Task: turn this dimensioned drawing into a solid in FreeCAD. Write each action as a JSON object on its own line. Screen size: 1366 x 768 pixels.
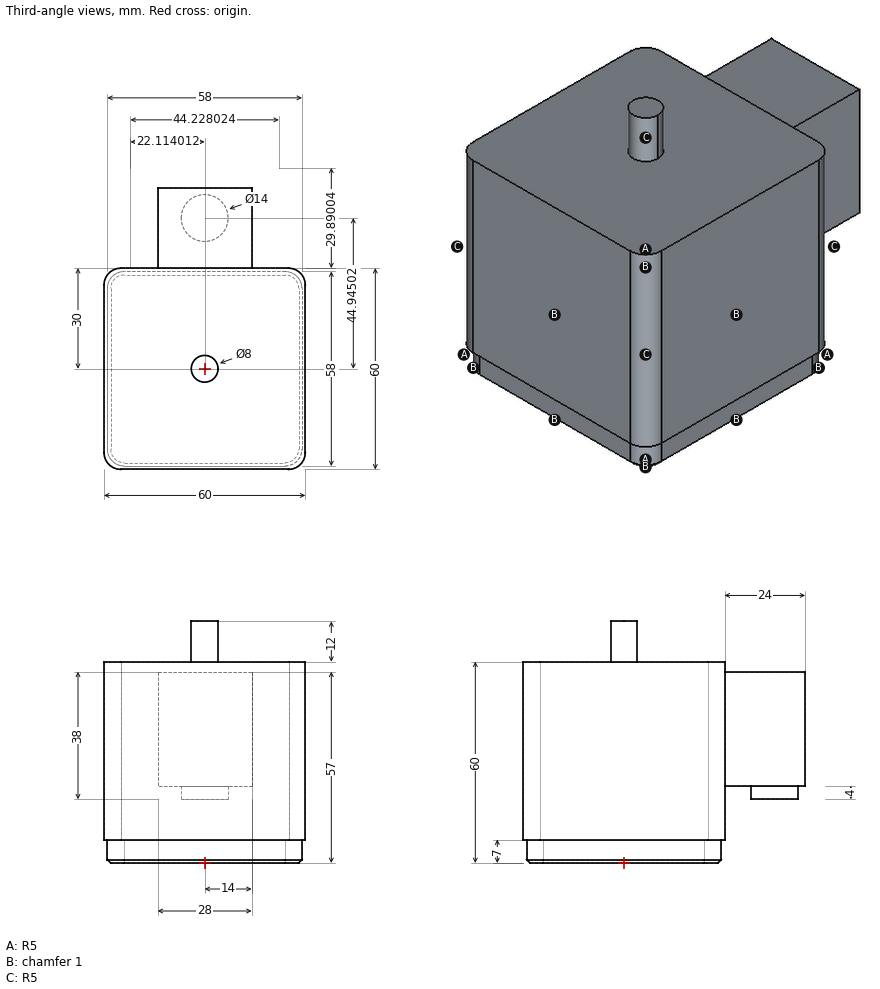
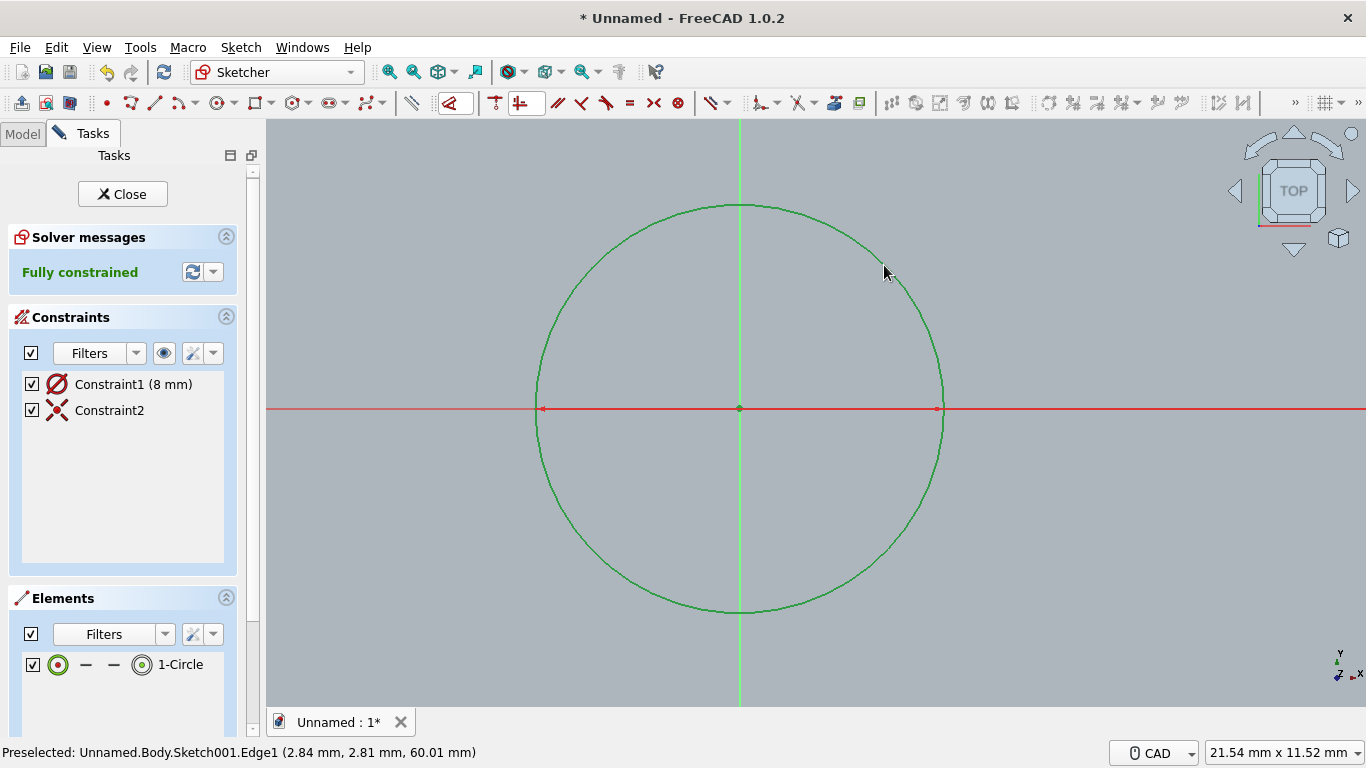
{"action": "left_click", "coordinate": [123, 194]}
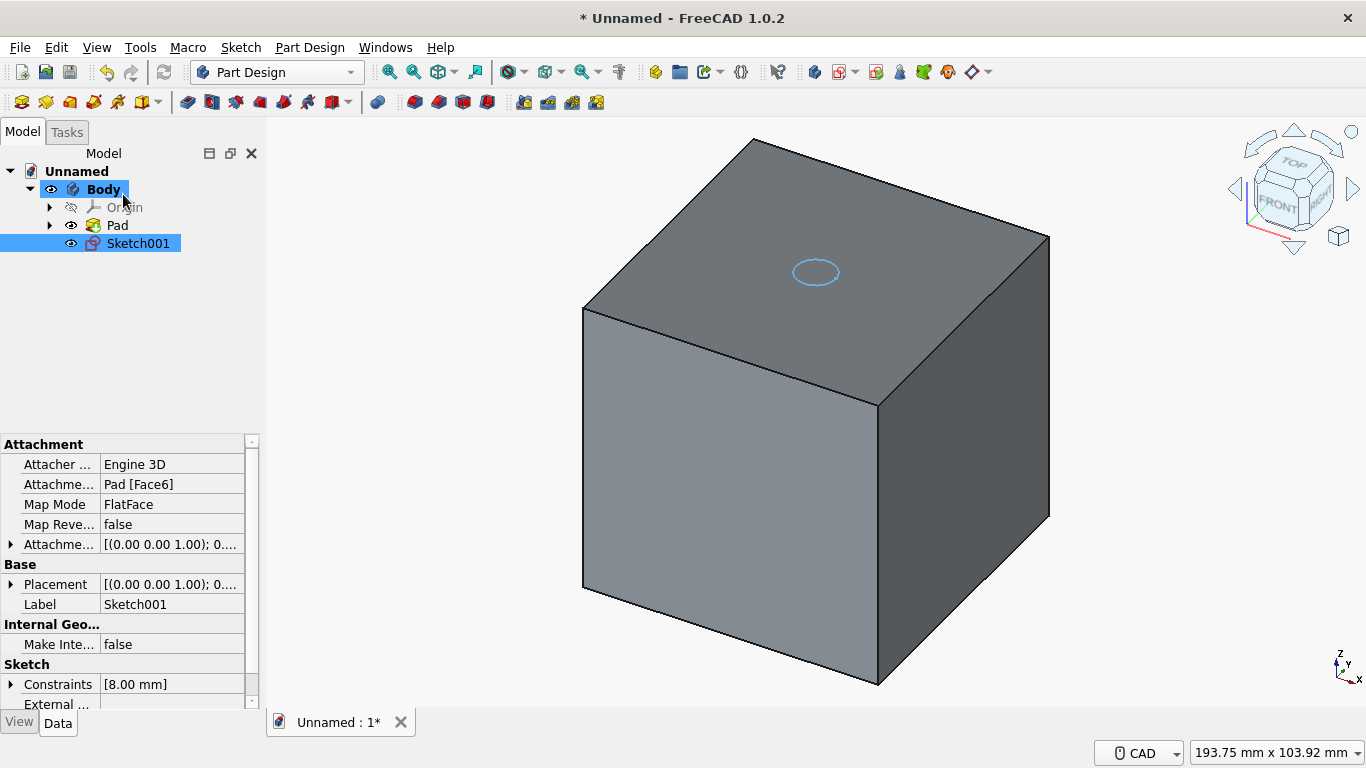
{"action": "left_click", "coordinate": [22, 102]}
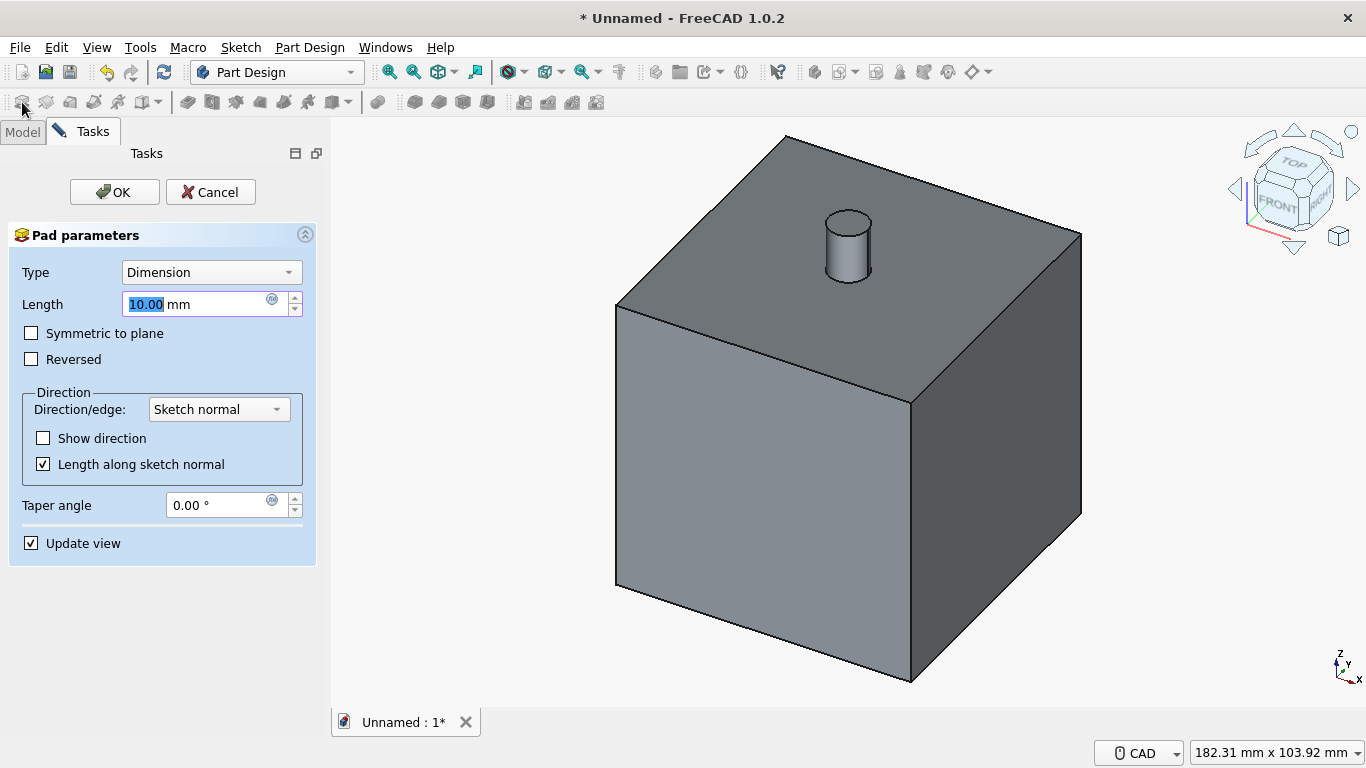
{"action": "type", "text": "12"}
{"action": "key", "text": "Tab"}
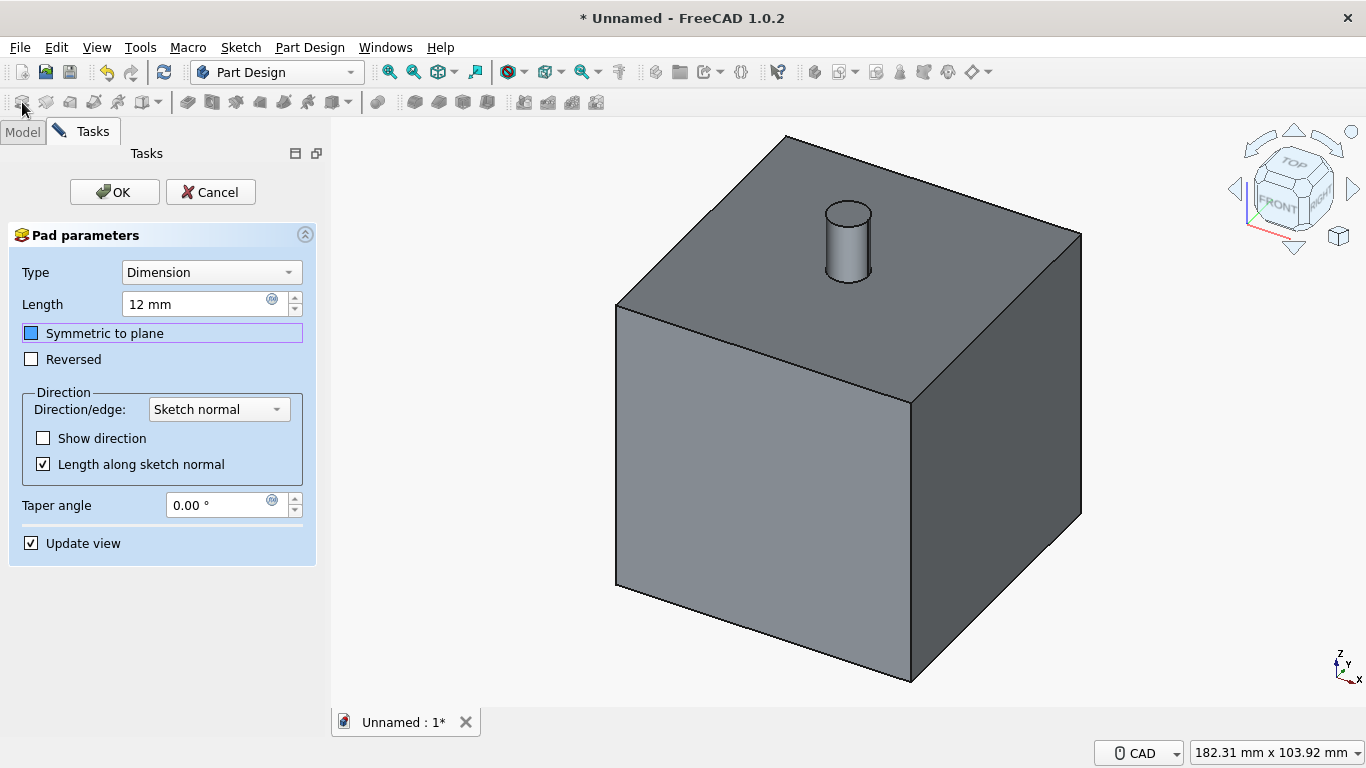
{"action": "left_click", "coordinate": [115, 192]}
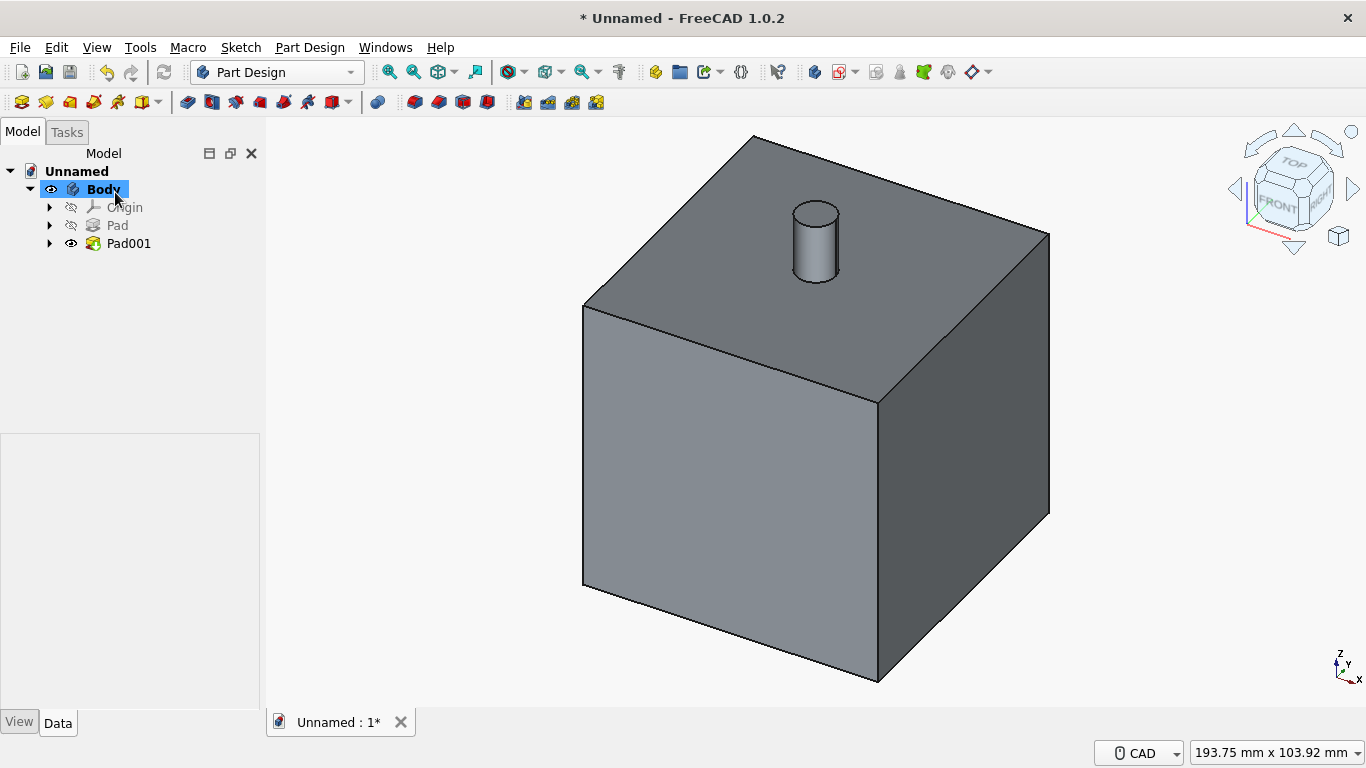
{"action": "left_click", "coordinate": [390, 72]}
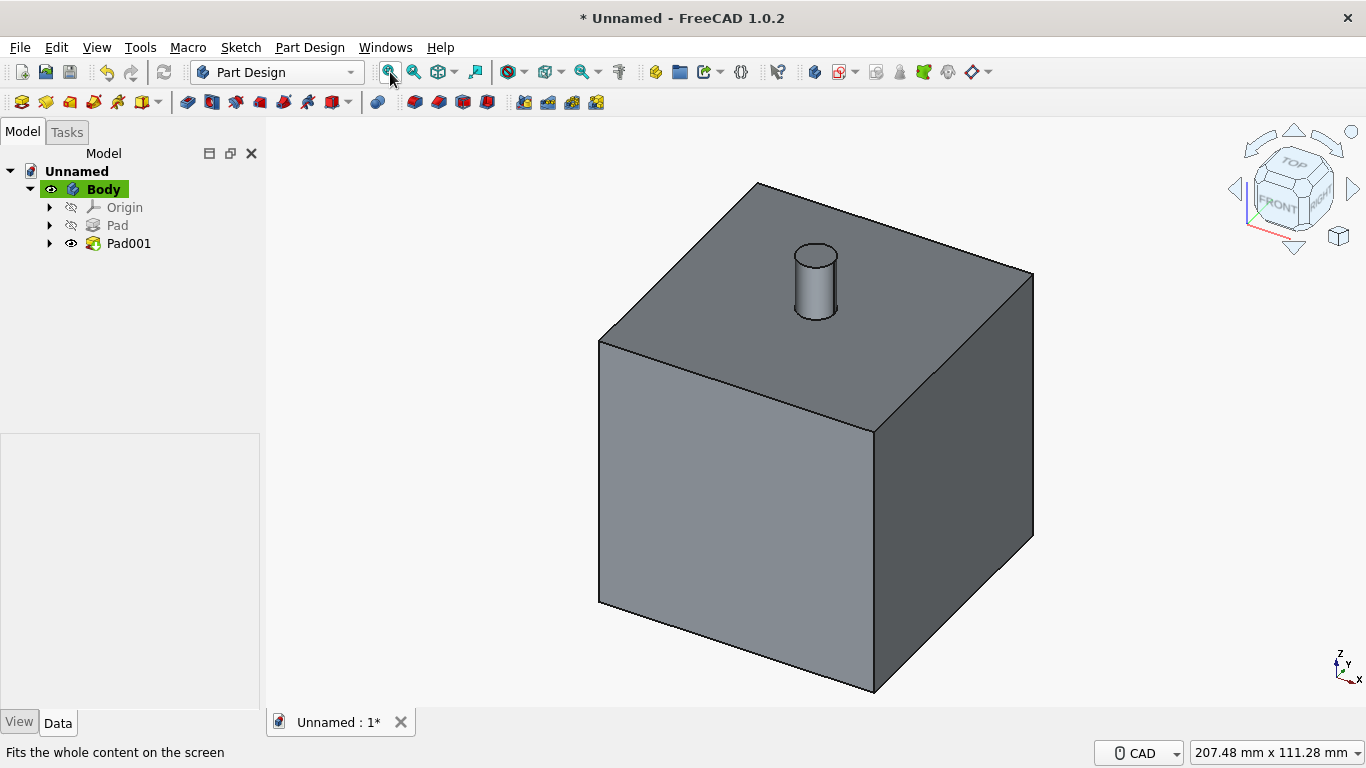
{"action": "key", "text": "5"}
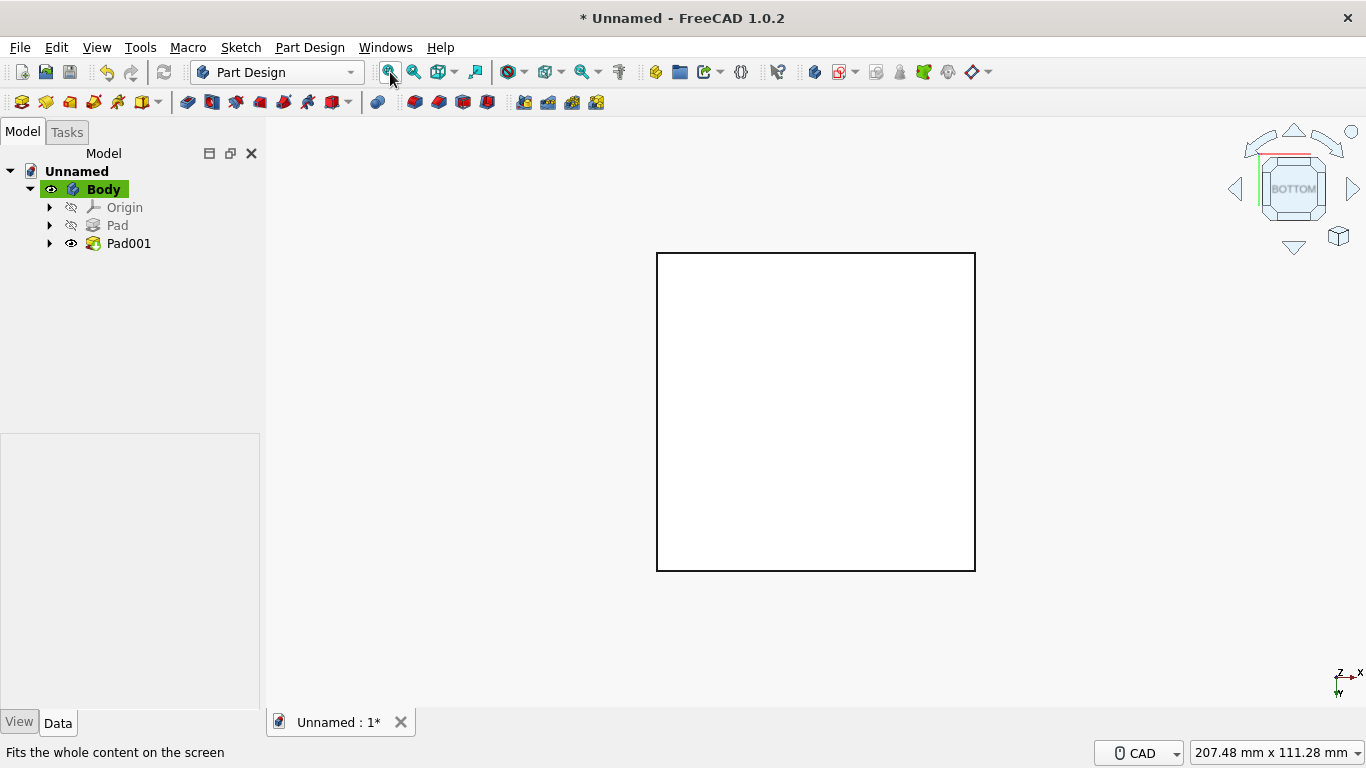
{"action": "left_click", "coordinate": [816, 411]}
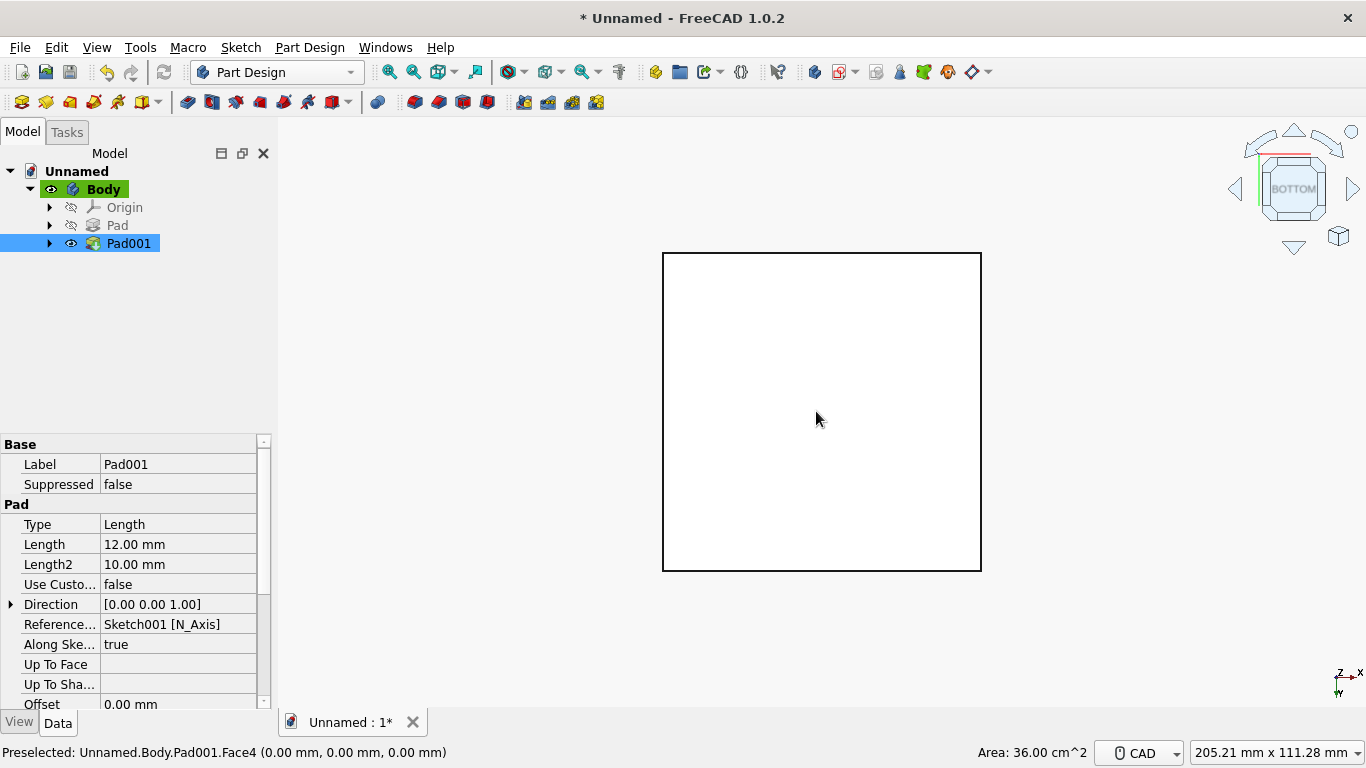
{"action": "left_click", "coordinate": [840, 72]}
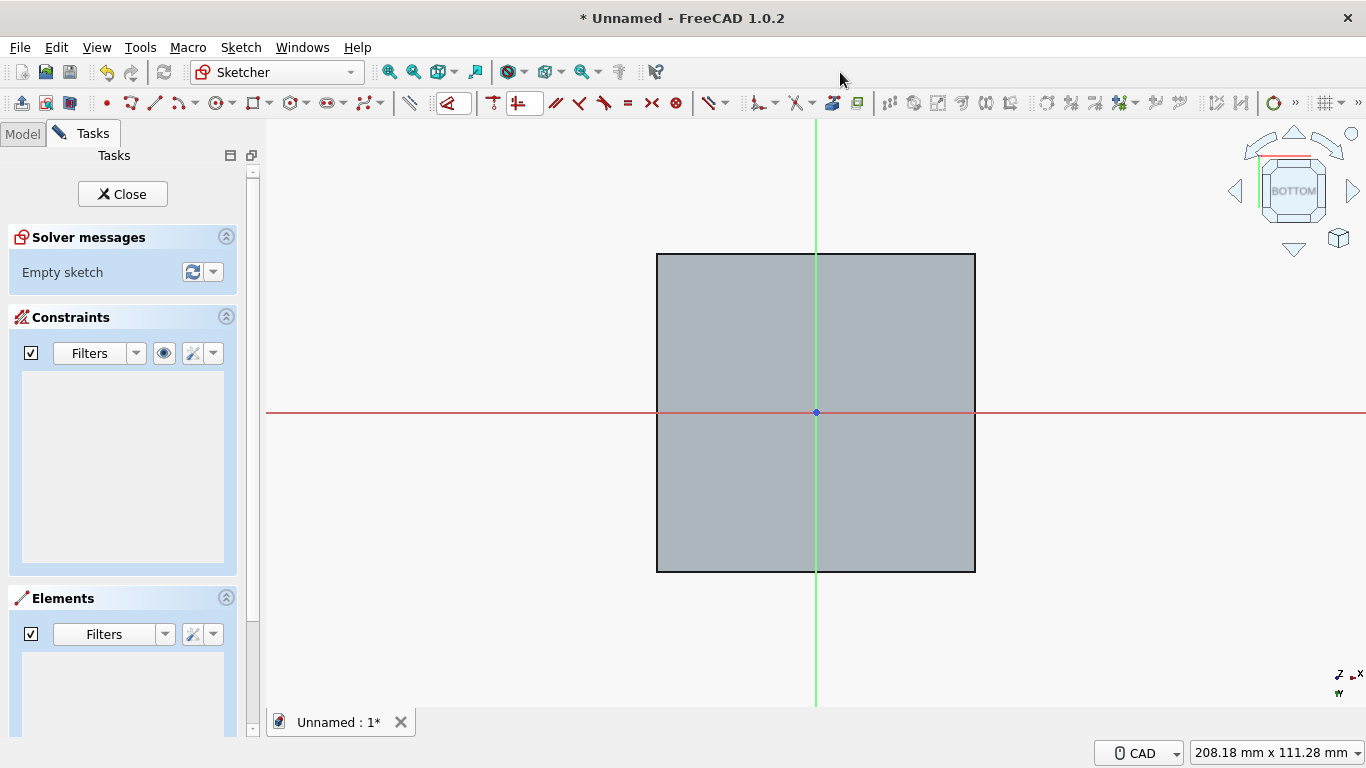
{"action": "key", "text": "g v"}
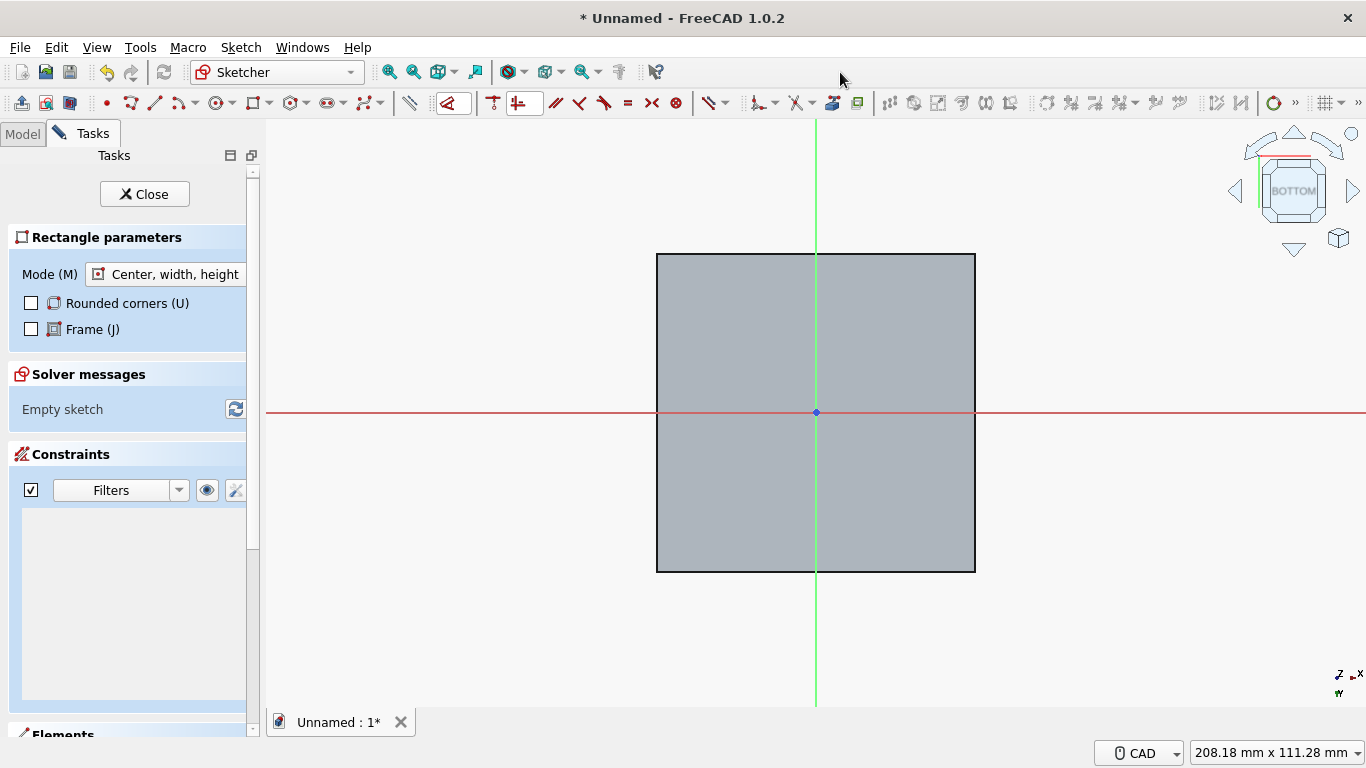
{"action": "left_click", "coordinate": [816, 413]}
{"action": "mouse_move", "coordinate": [975, 254]}